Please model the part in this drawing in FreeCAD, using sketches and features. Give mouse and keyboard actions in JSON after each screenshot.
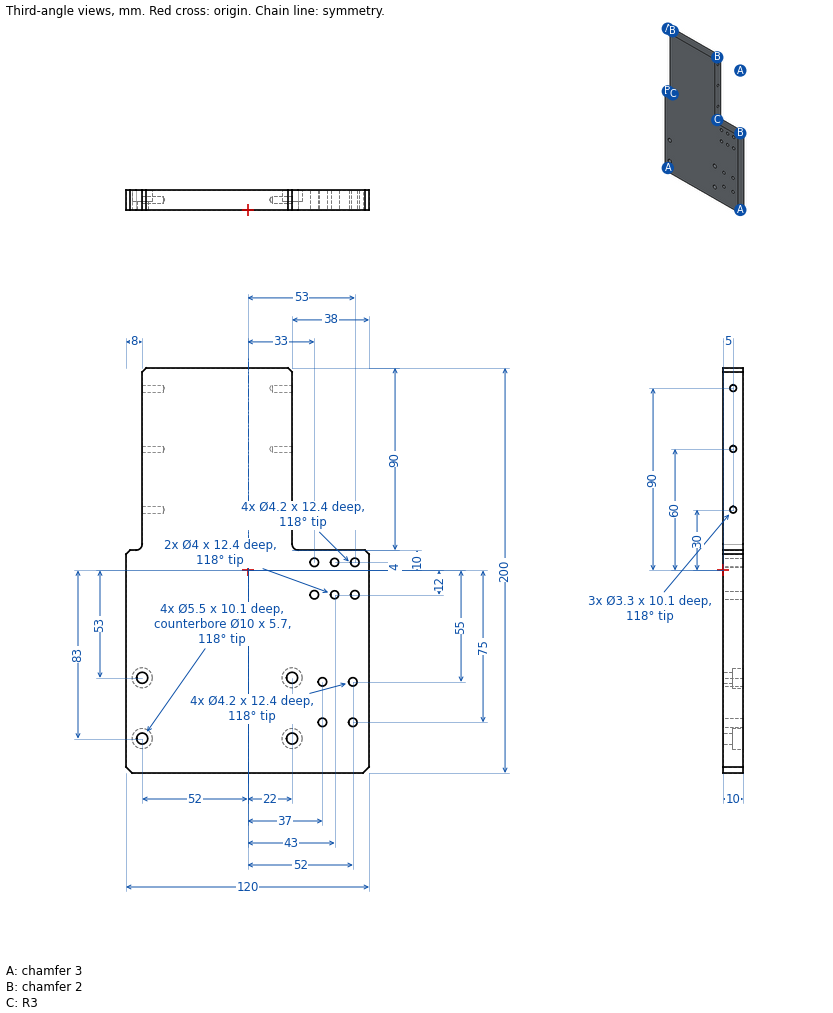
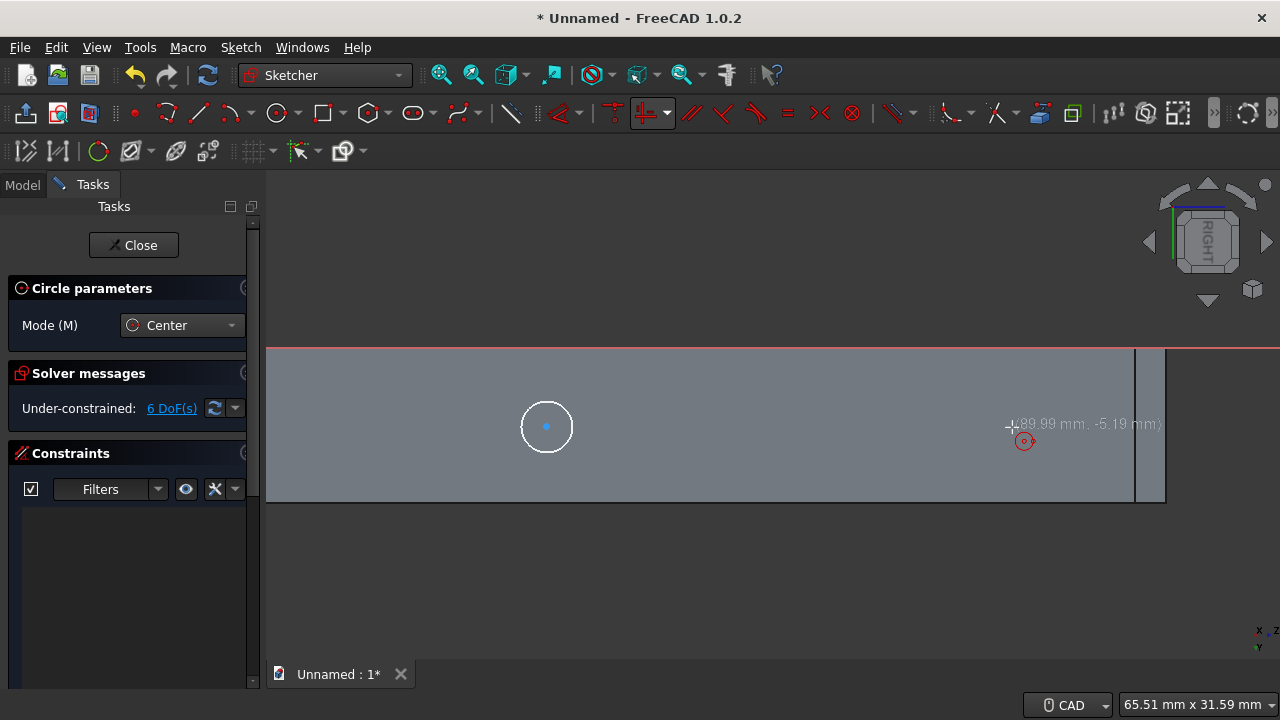
{"action": "left_click", "coordinate": [1011, 426]}
{"action": "left_click", "coordinate": [1029, 408]}
{"action": "key", "text": "Escape"}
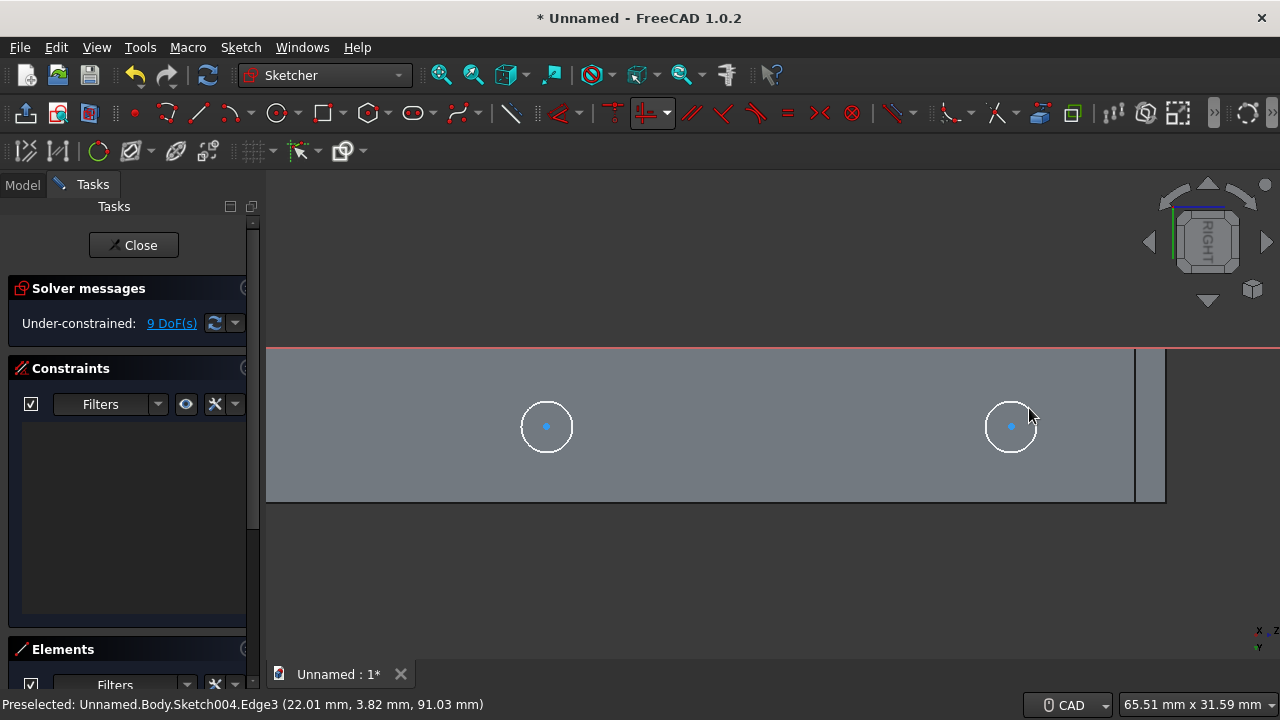
{"action": "scroll", "coordinate": [1012, 427], "scroll_direction": "down", "scroll_amount": 4}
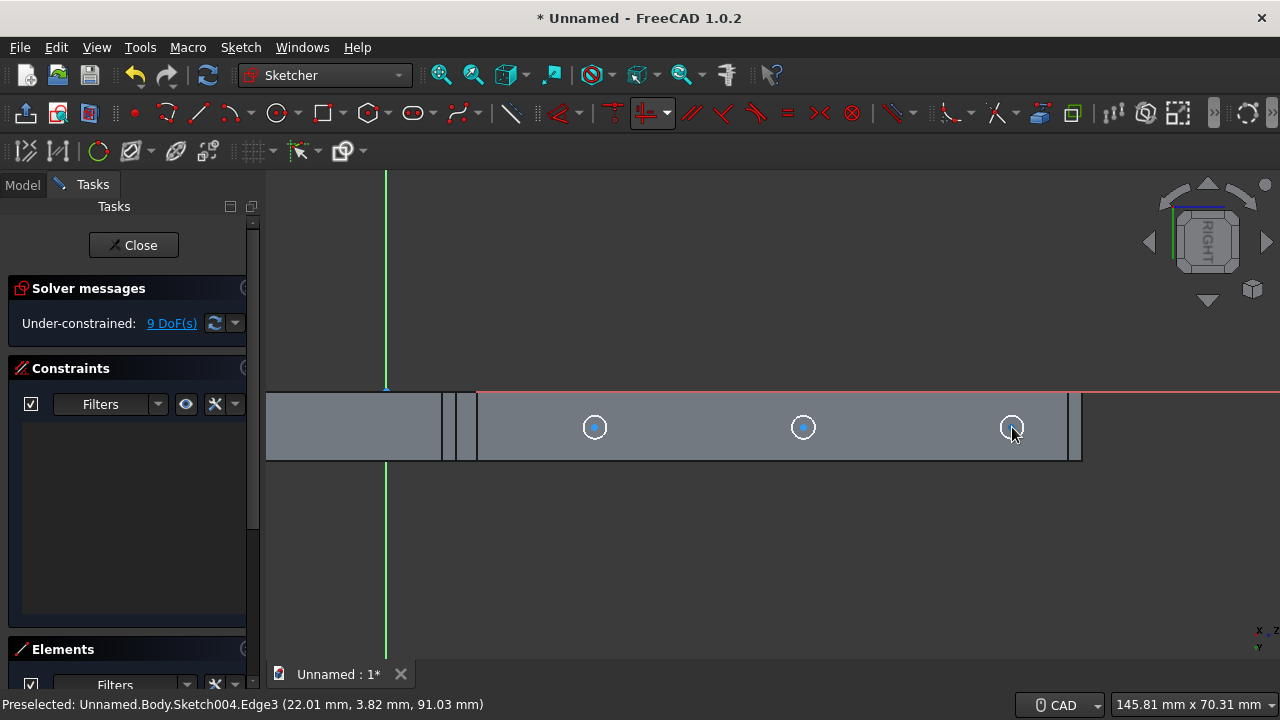
{"action": "left_click", "coordinate": [603, 419]}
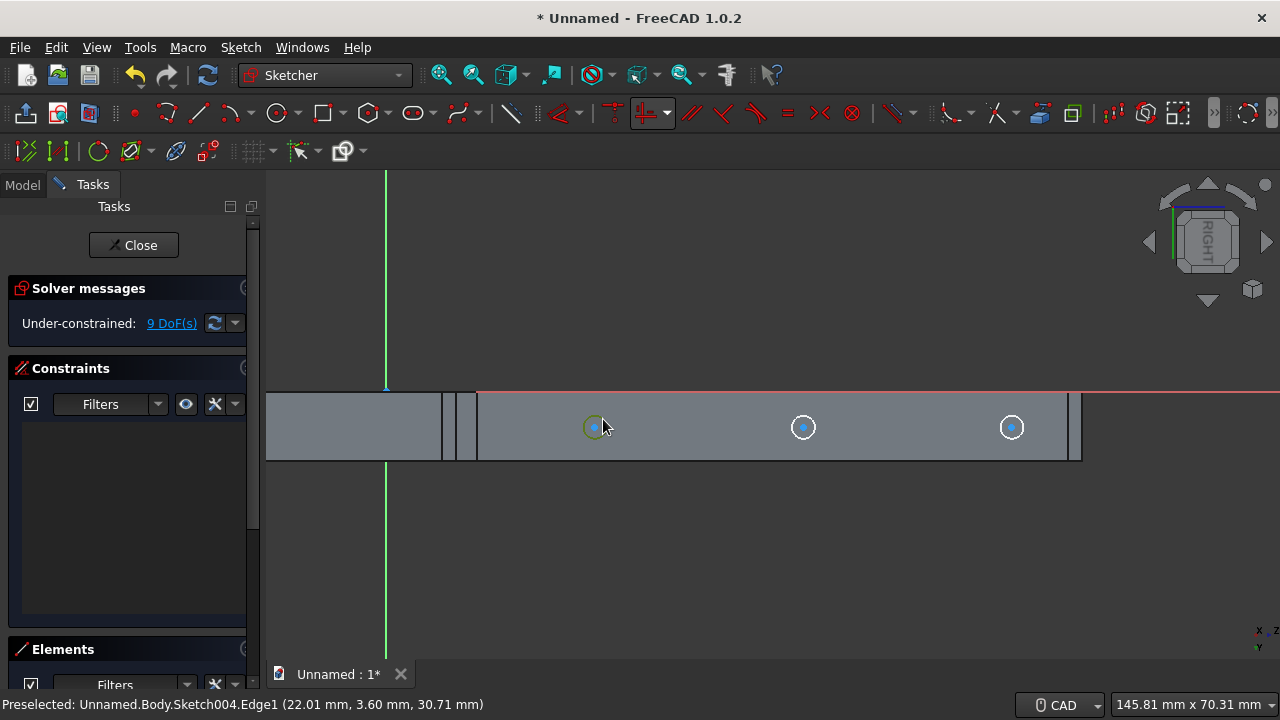
{"action": "left_click", "coordinate": [811, 419]}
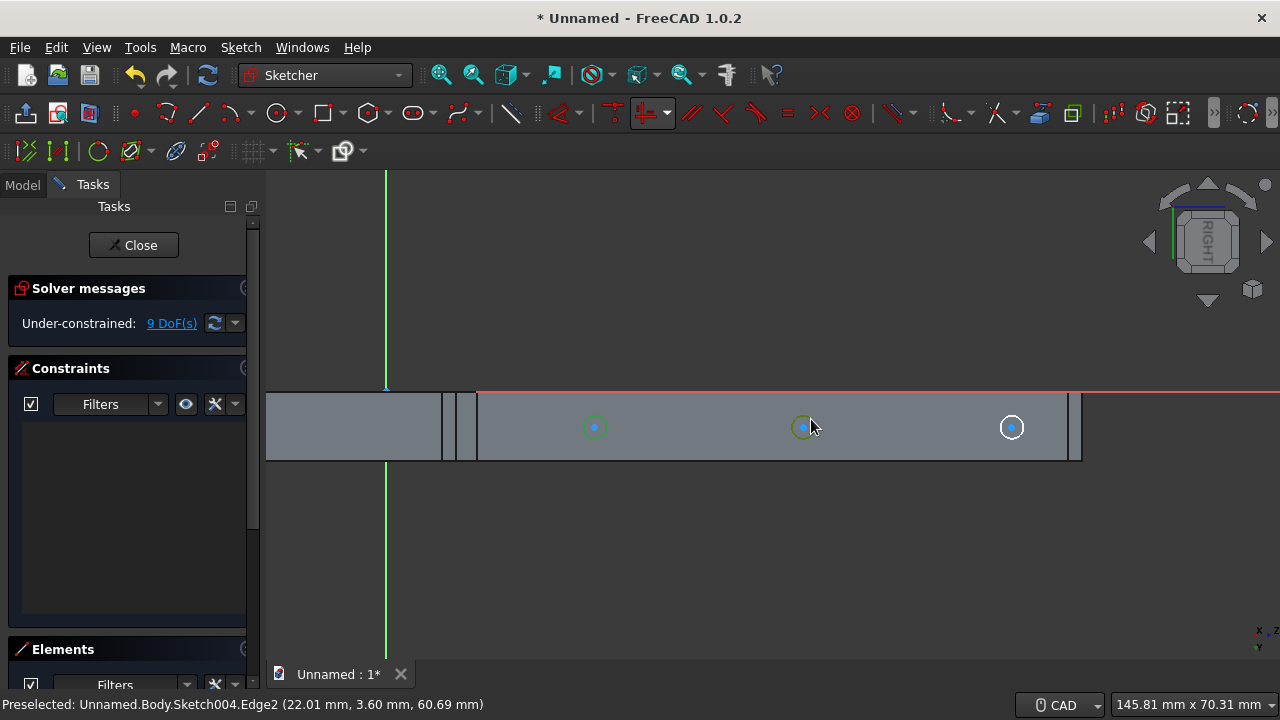
{"action": "left_click", "coordinate": [1020, 419]}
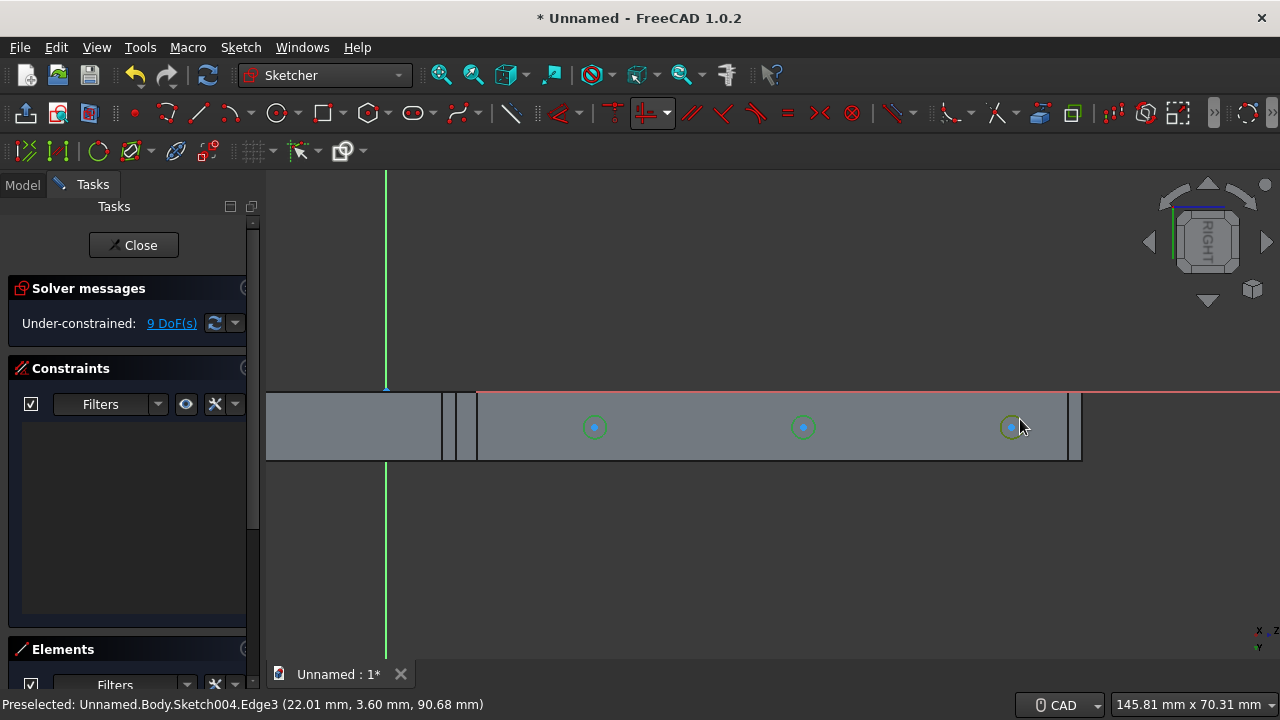
{"action": "left_click", "coordinate": [788, 114]}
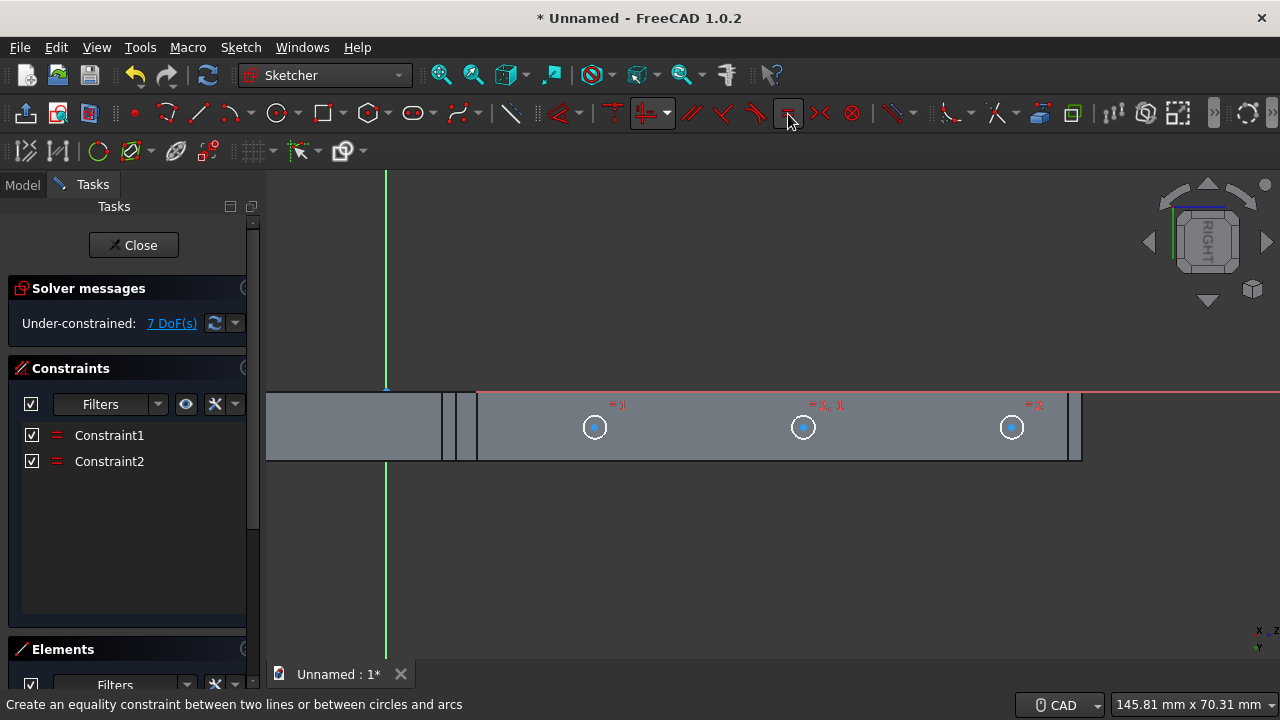
{"action": "left_click", "coordinate": [595, 427]}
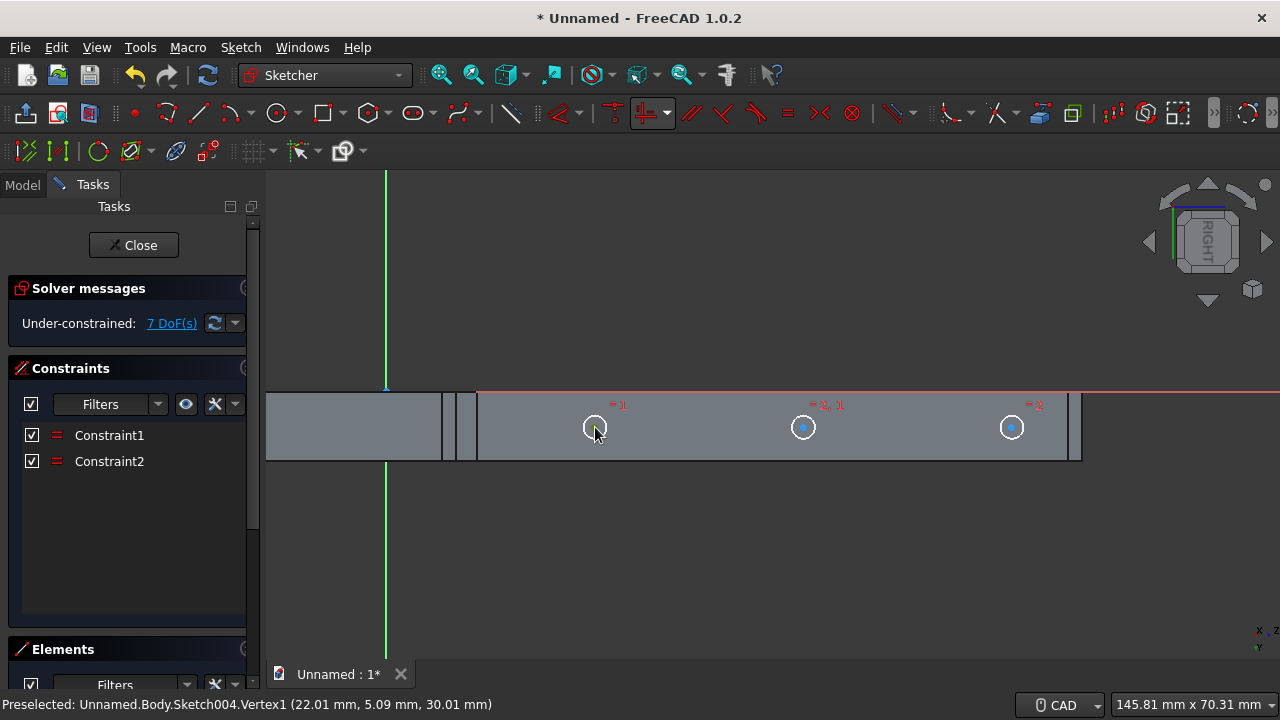
{"action": "left_click", "coordinate": [803, 427]}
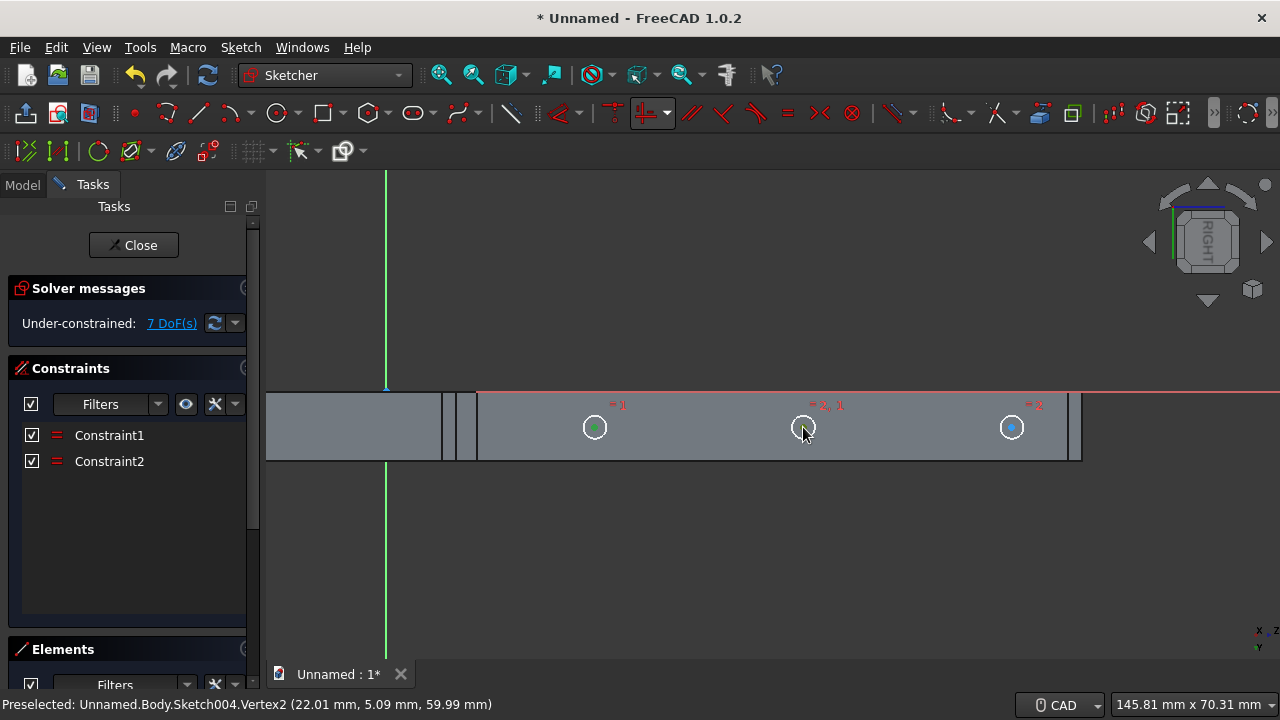
{"action": "key", "text": "h"}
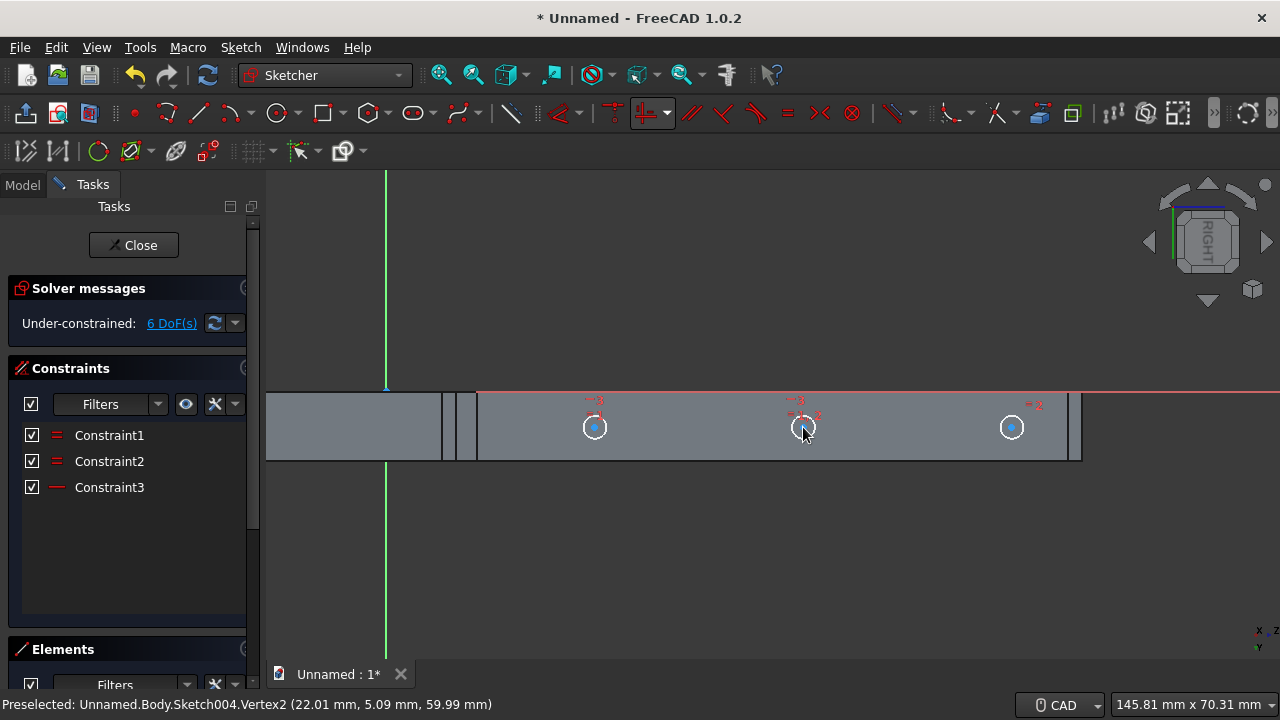
{"action": "left_click", "coordinate": [803, 427]}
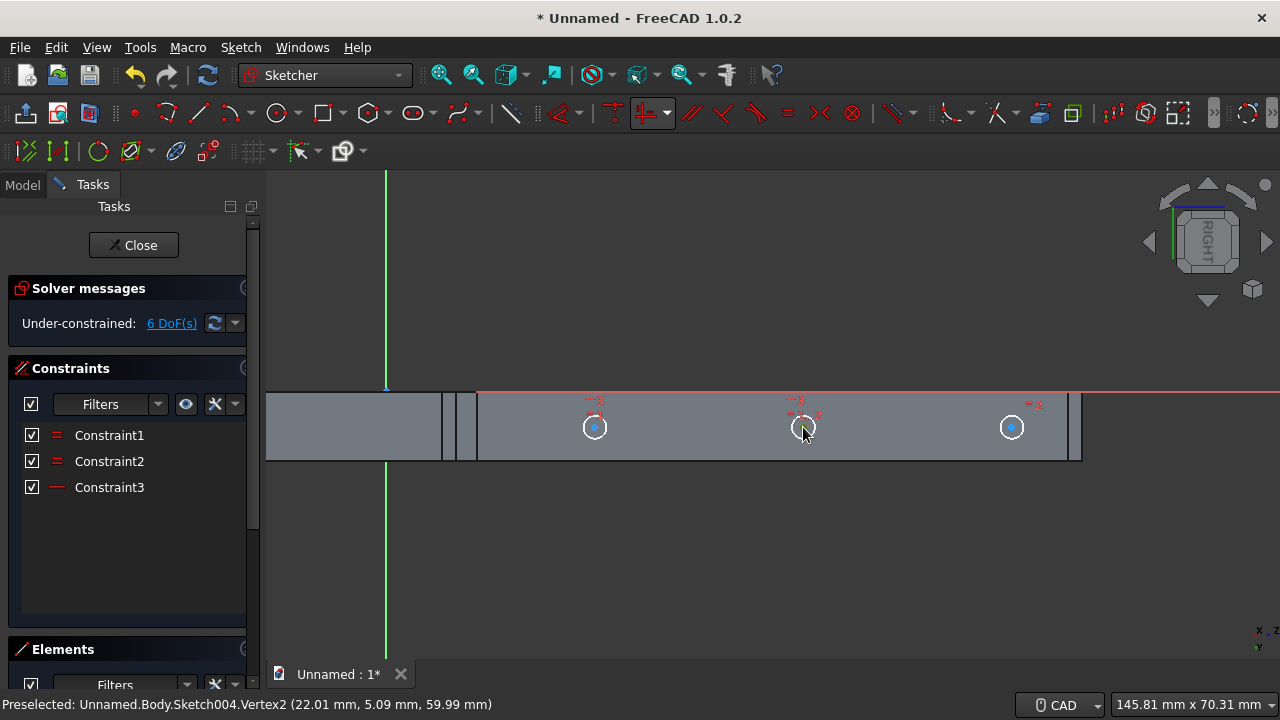
{"action": "left_click", "coordinate": [1012, 427]}